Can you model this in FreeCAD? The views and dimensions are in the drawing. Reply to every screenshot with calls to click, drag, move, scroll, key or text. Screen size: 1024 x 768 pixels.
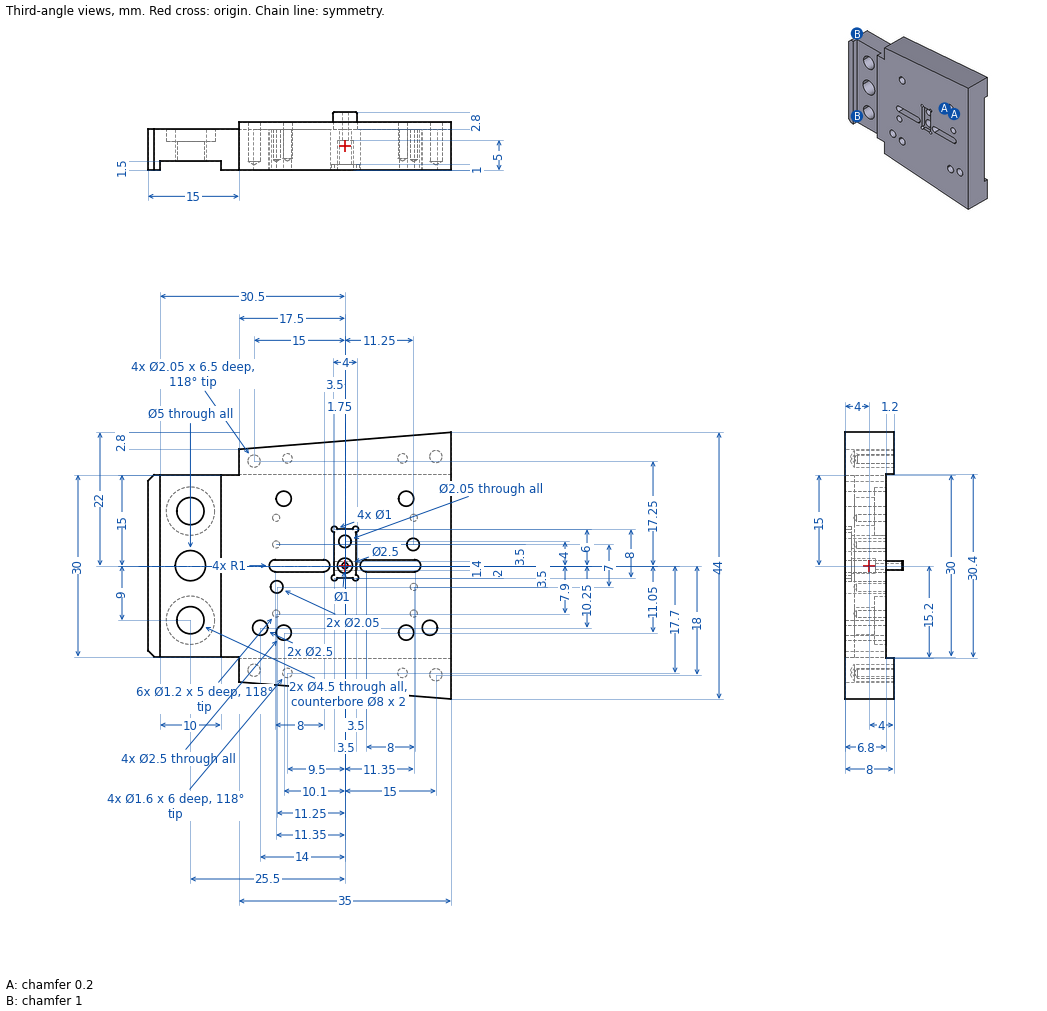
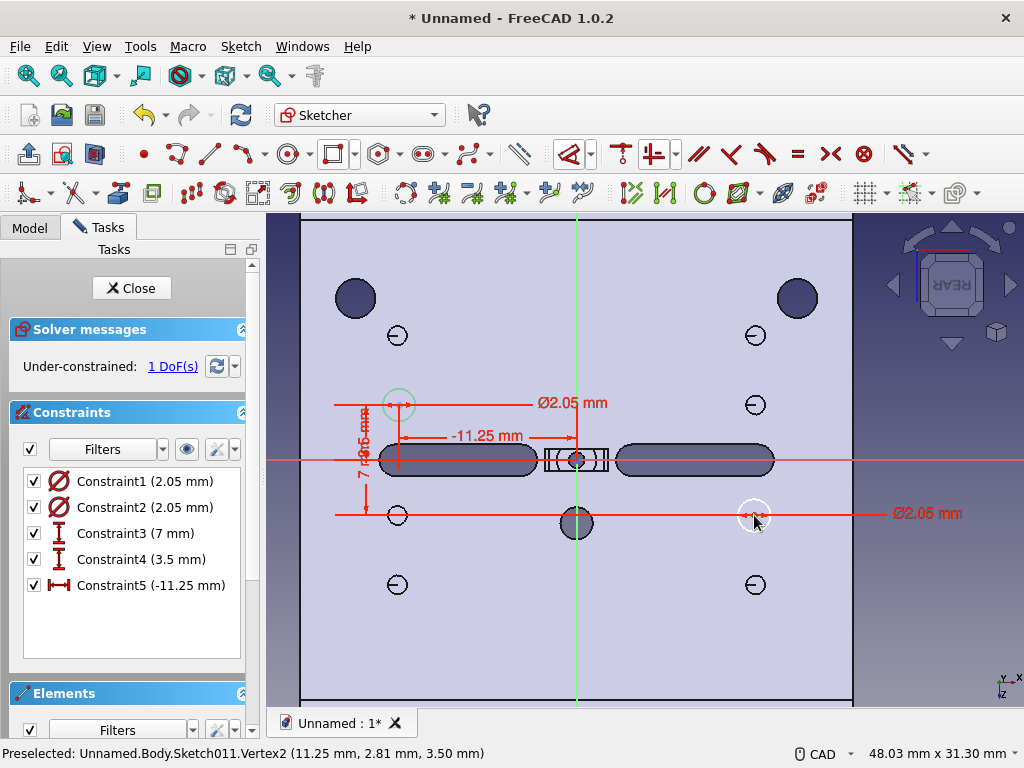
key(l)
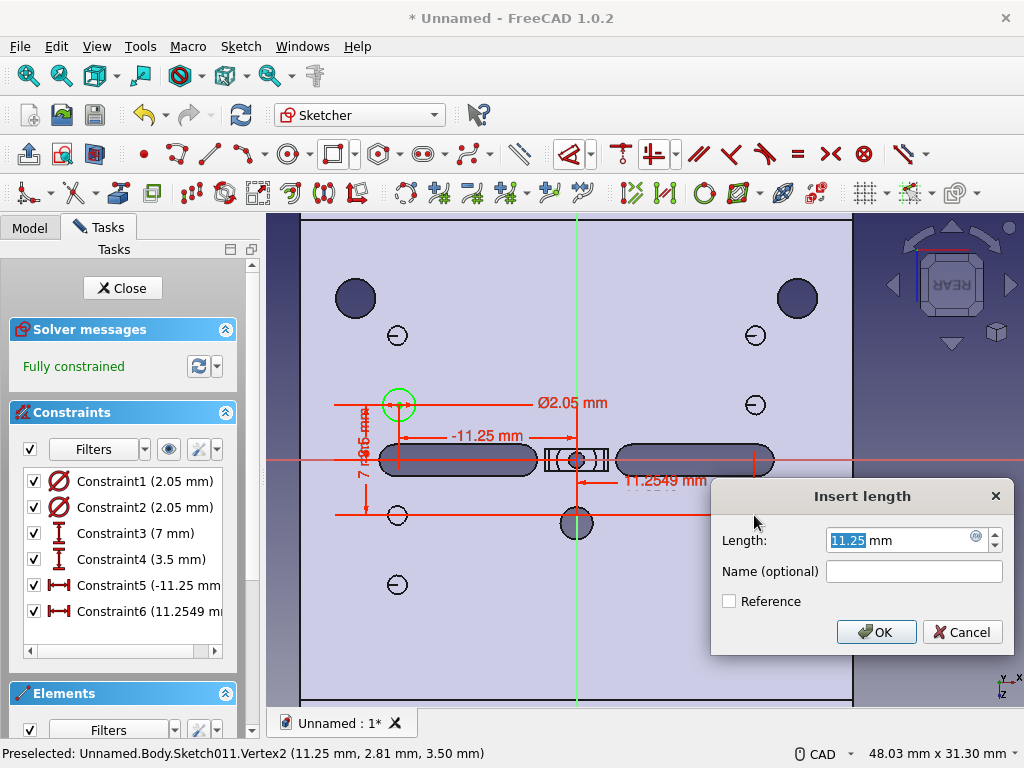
text(11.25)
key(Return)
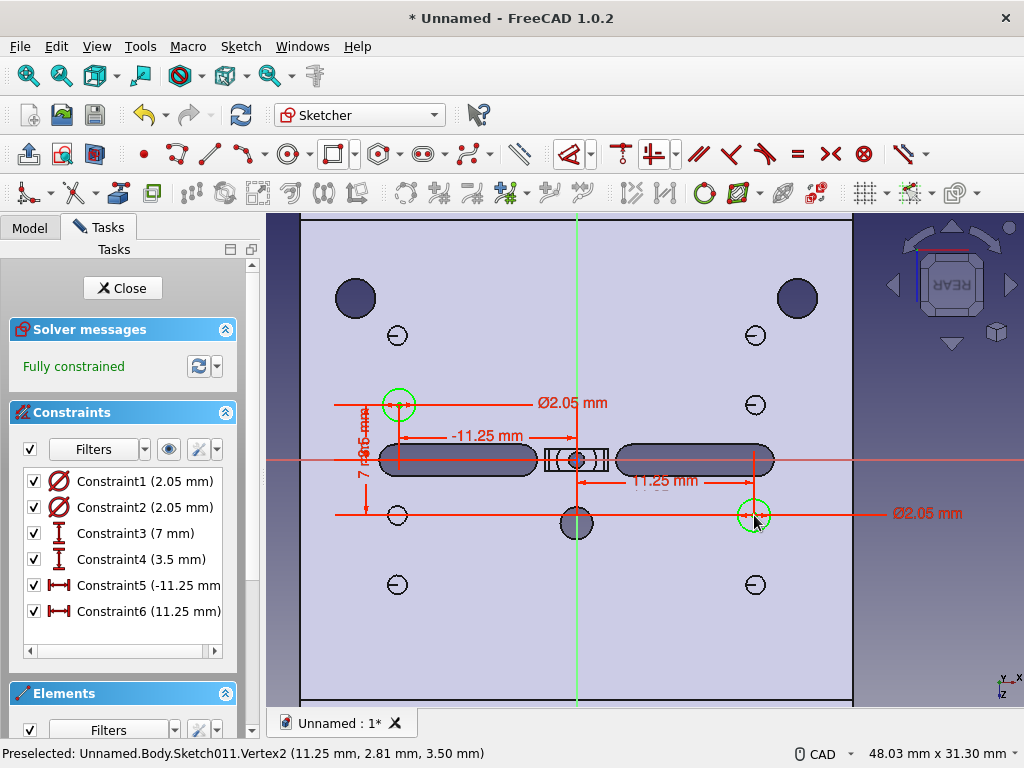
click(123, 288)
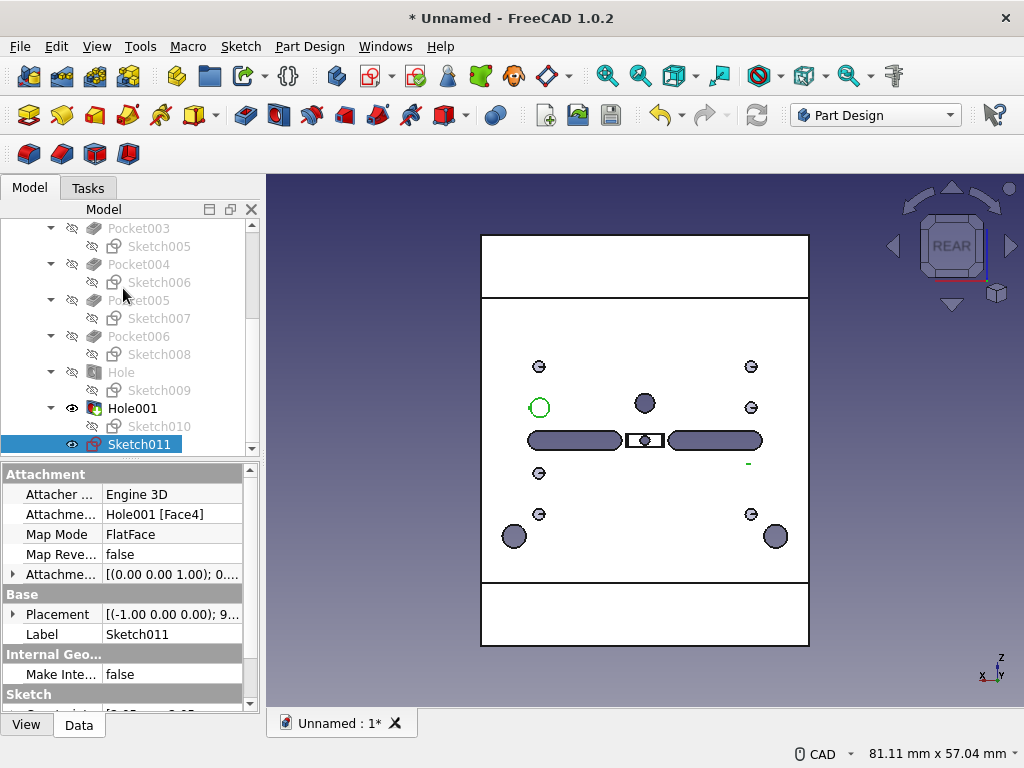
click(246, 116)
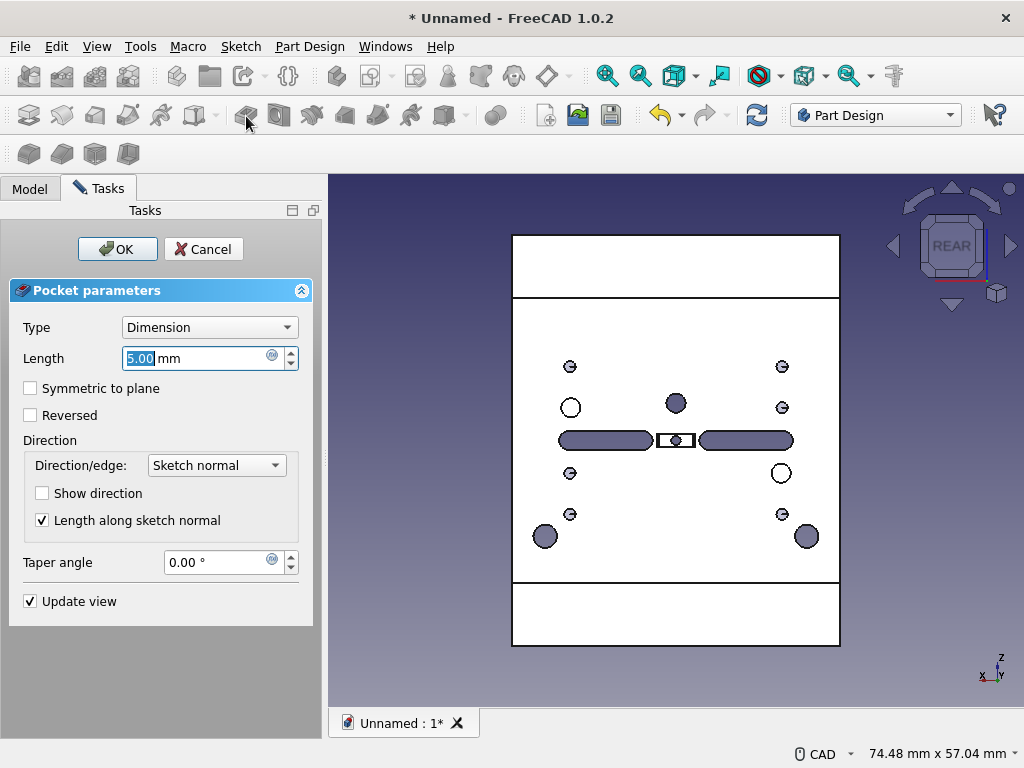
click(210, 328)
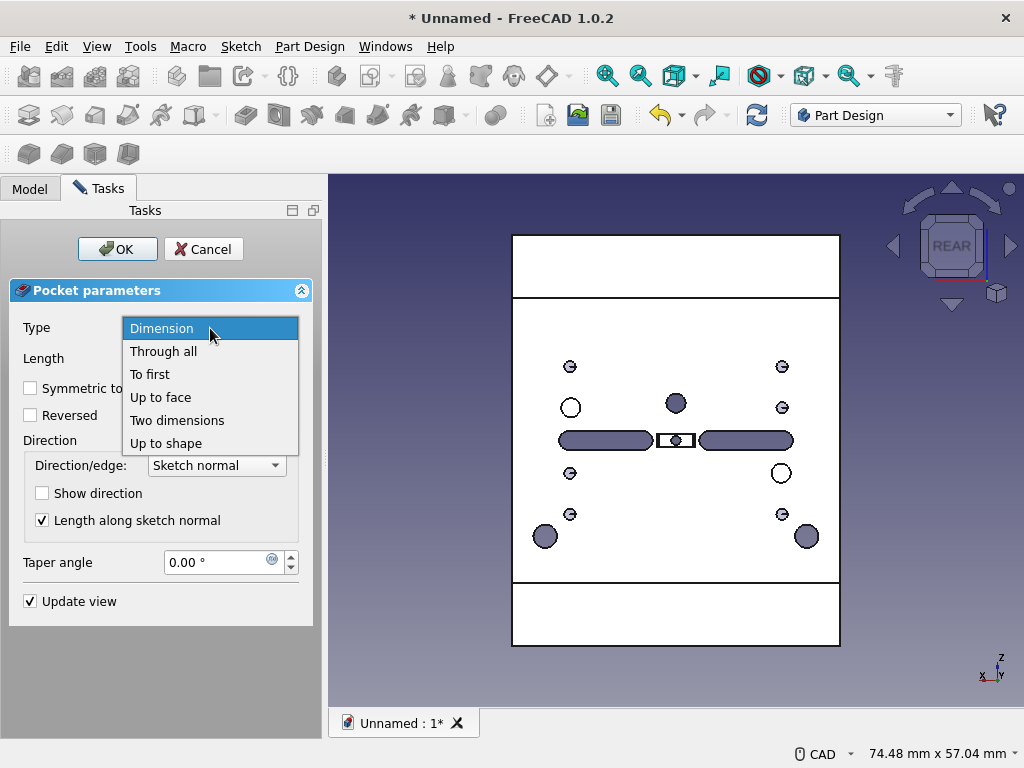
click(208, 352)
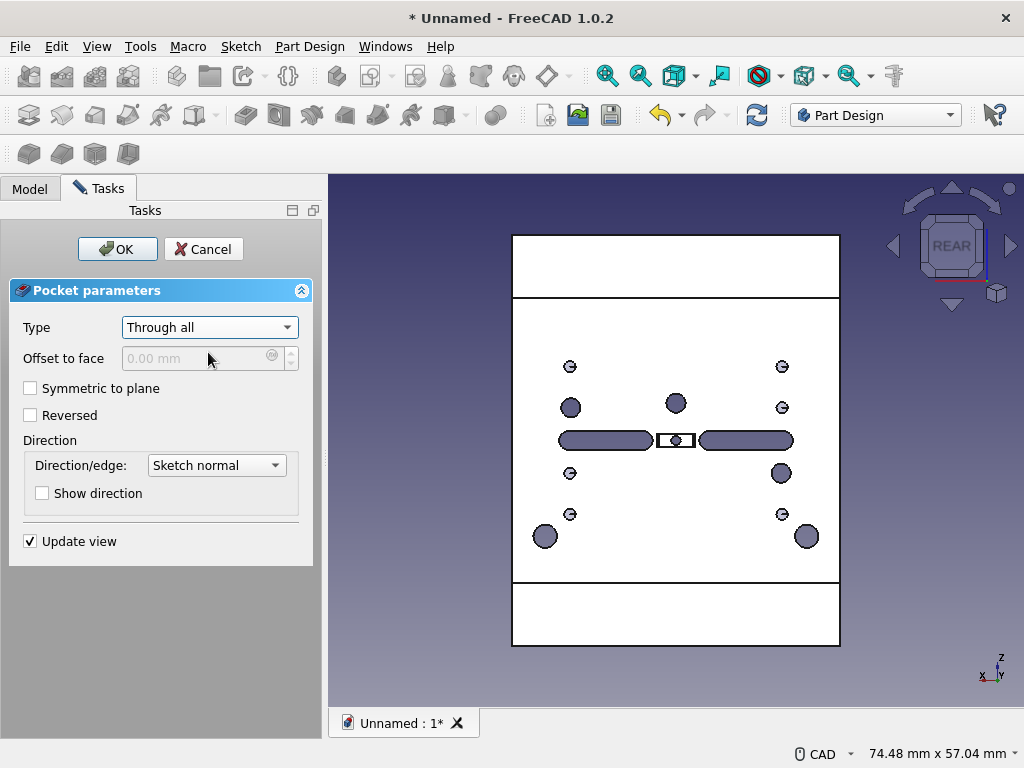
click(118, 249)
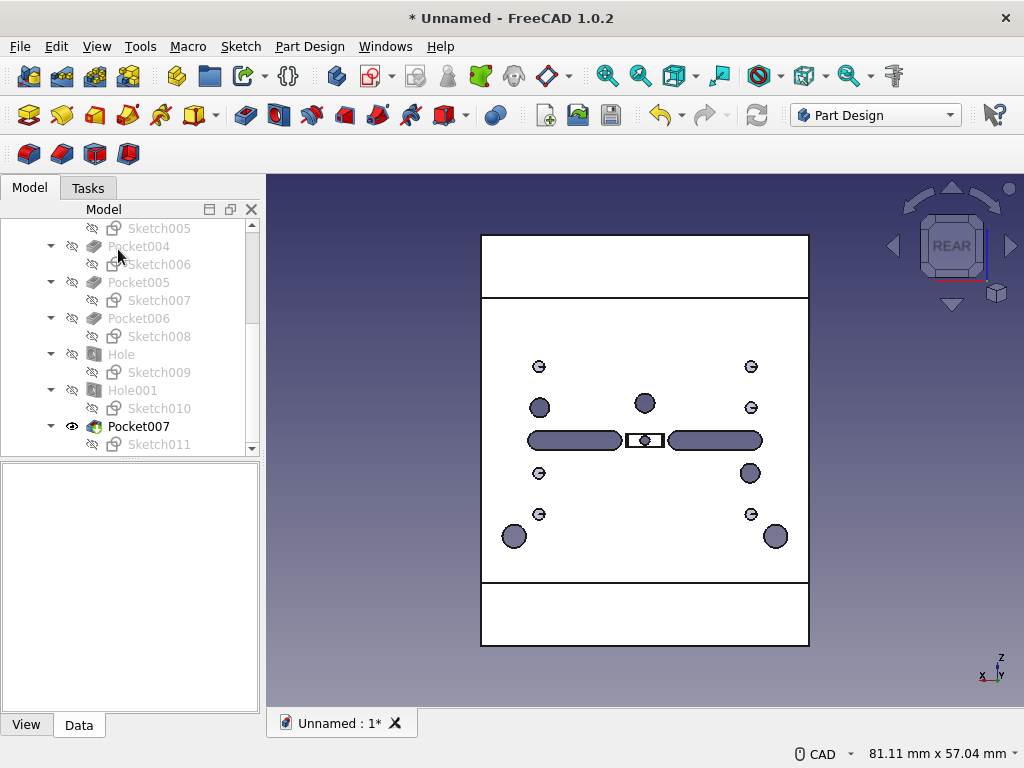
click(645, 521)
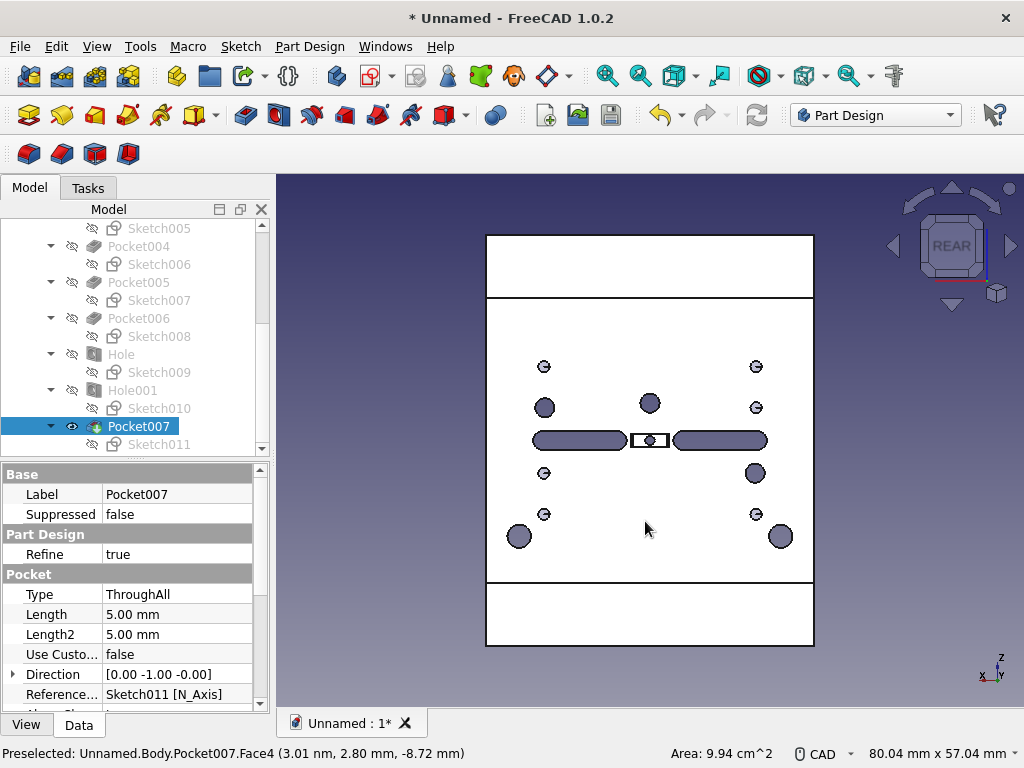
click(370, 76)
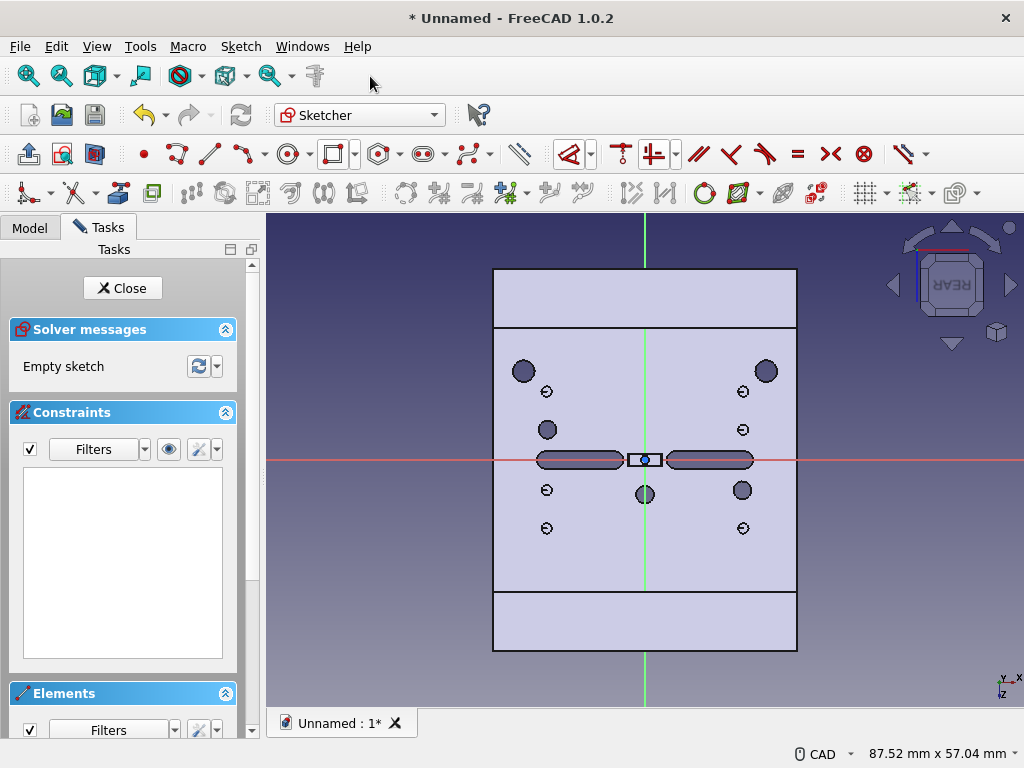
click(95, 154)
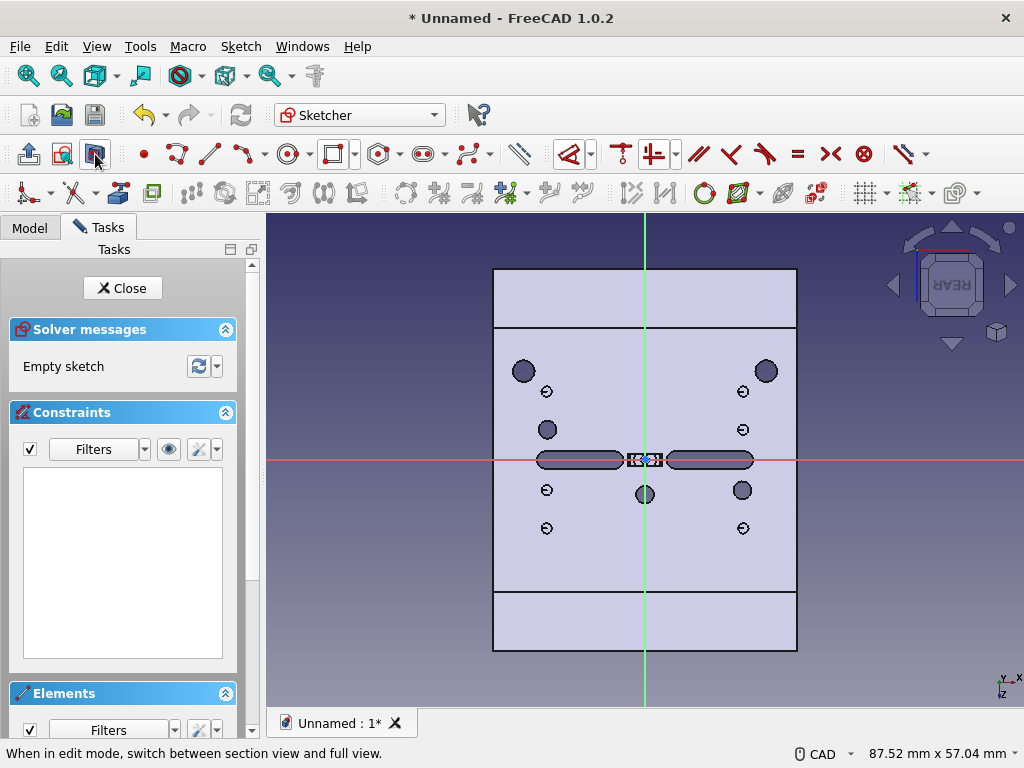
scroll(784, 460, up, 2)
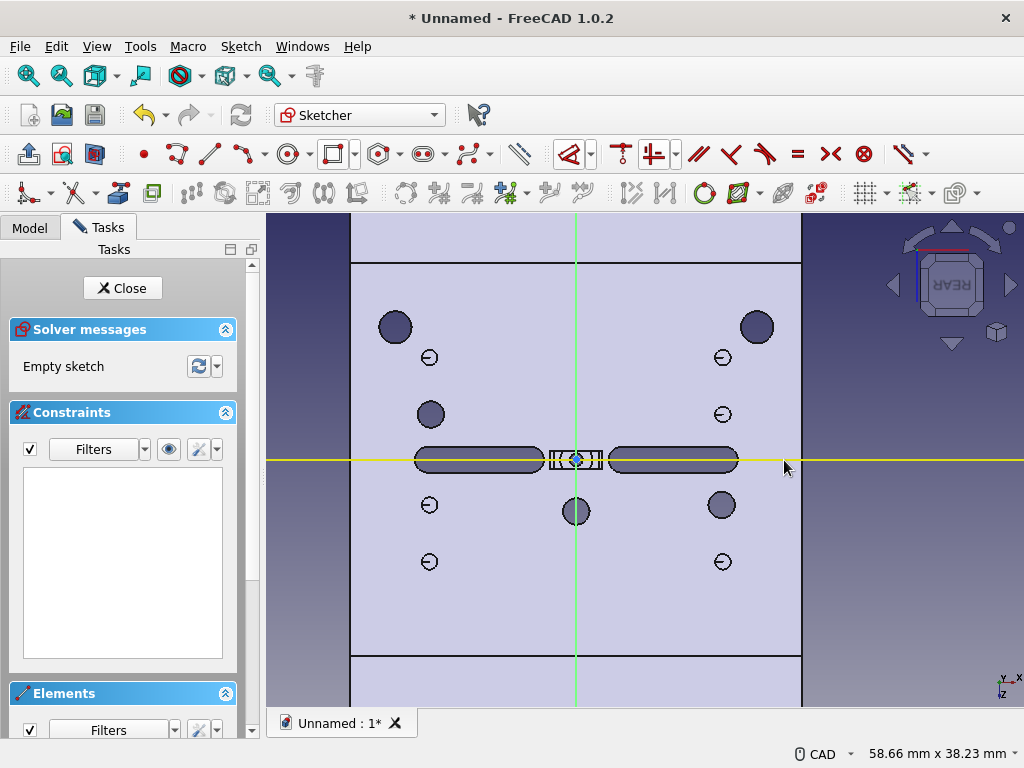
click(288, 154)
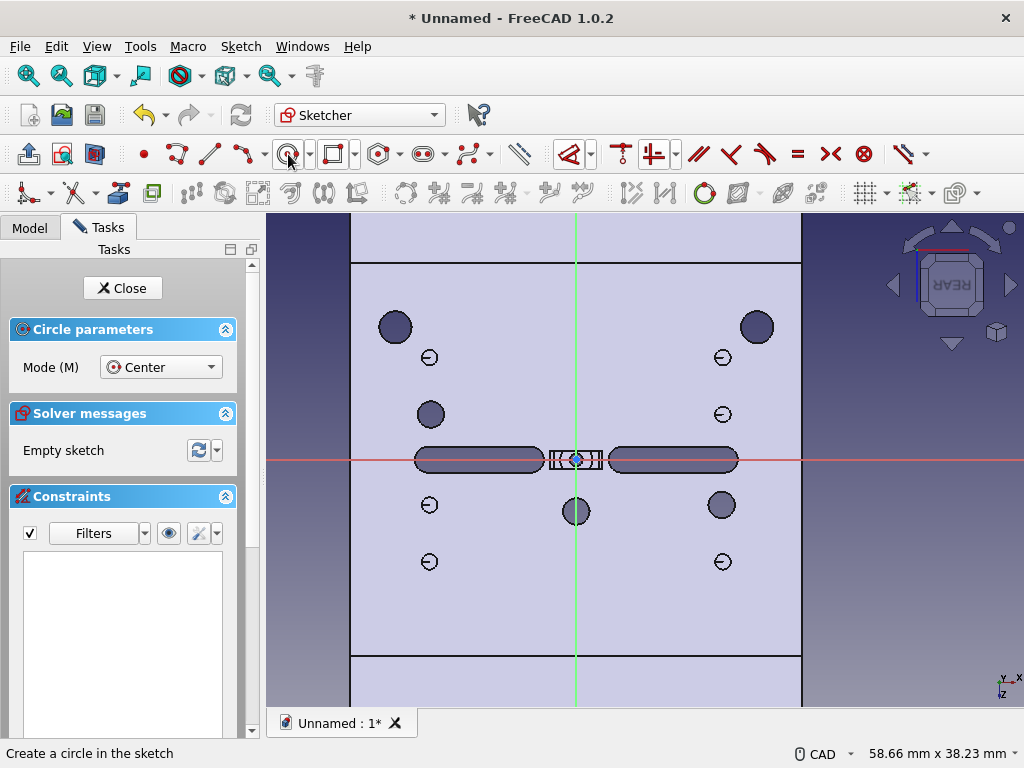
scroll(446, 317, up, 2)